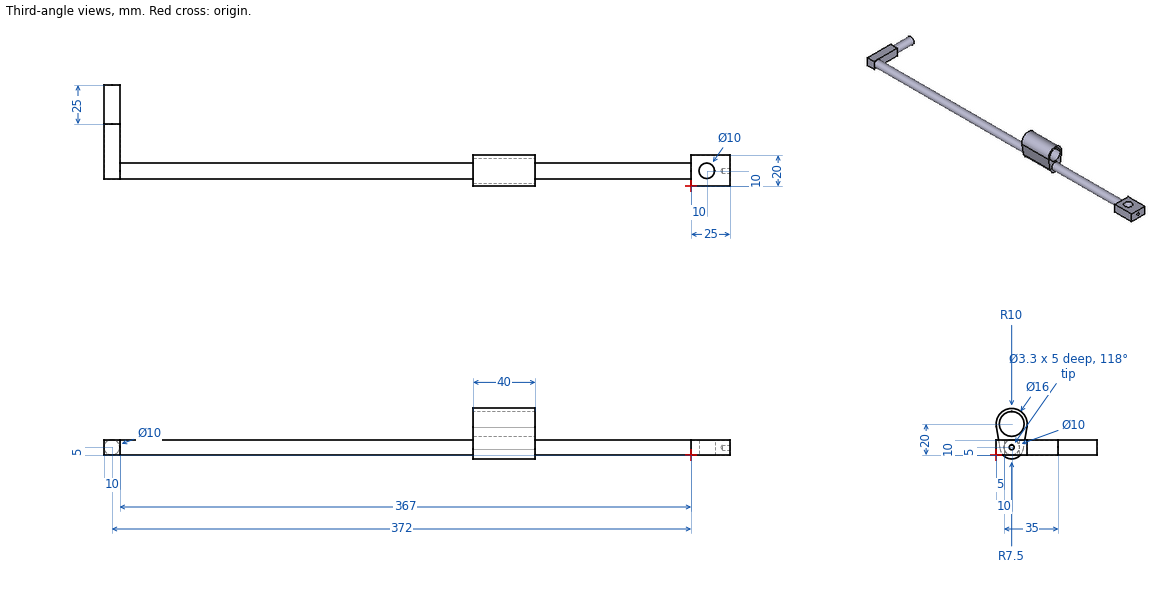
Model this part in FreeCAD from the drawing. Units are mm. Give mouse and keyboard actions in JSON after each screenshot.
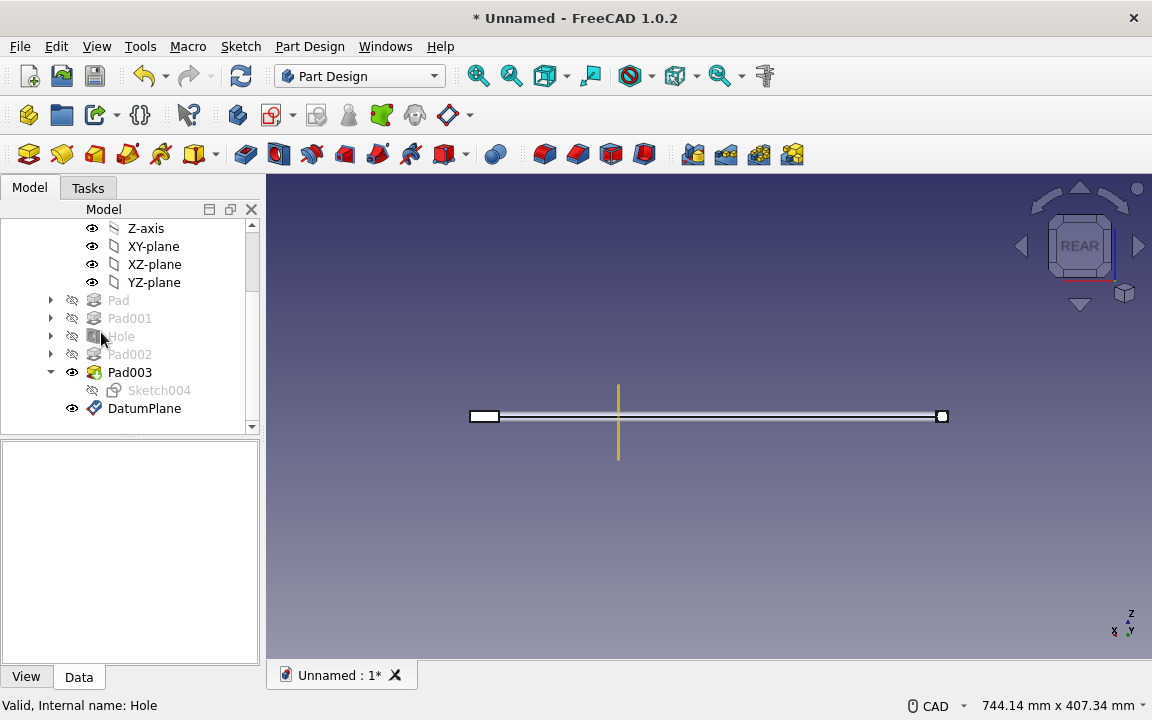
{"action": "left_click", "coordinate": [117, 408]}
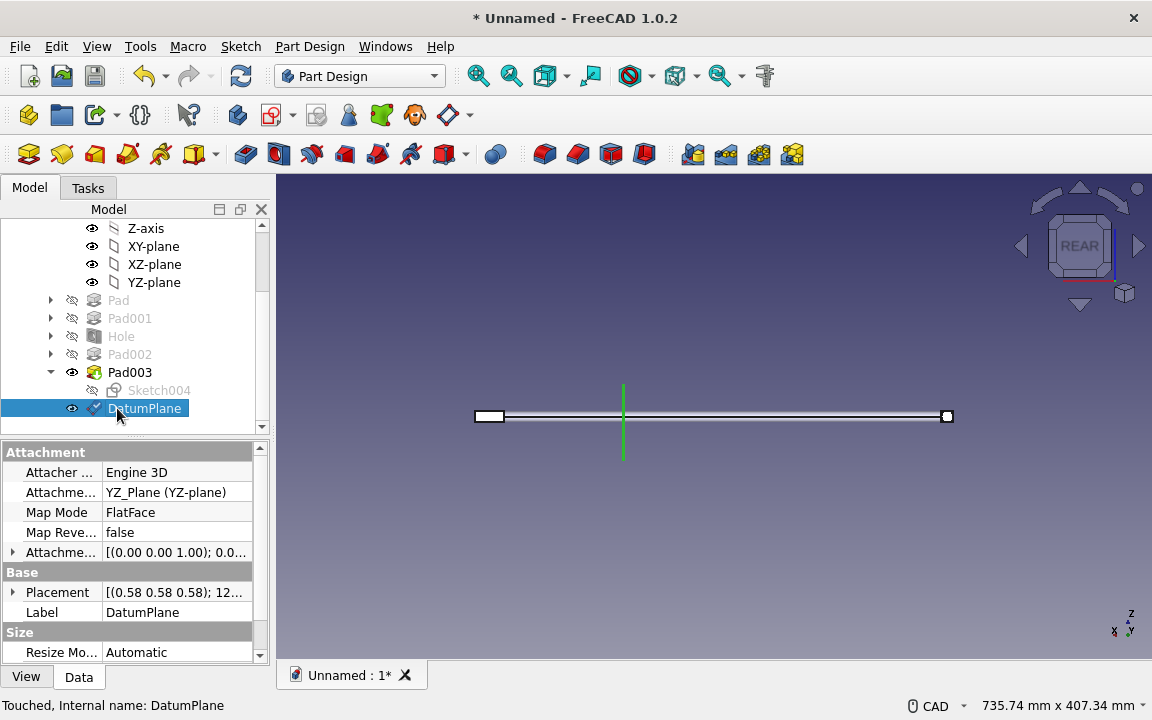
{"action": "left_click", "coordinate": [270, 116]}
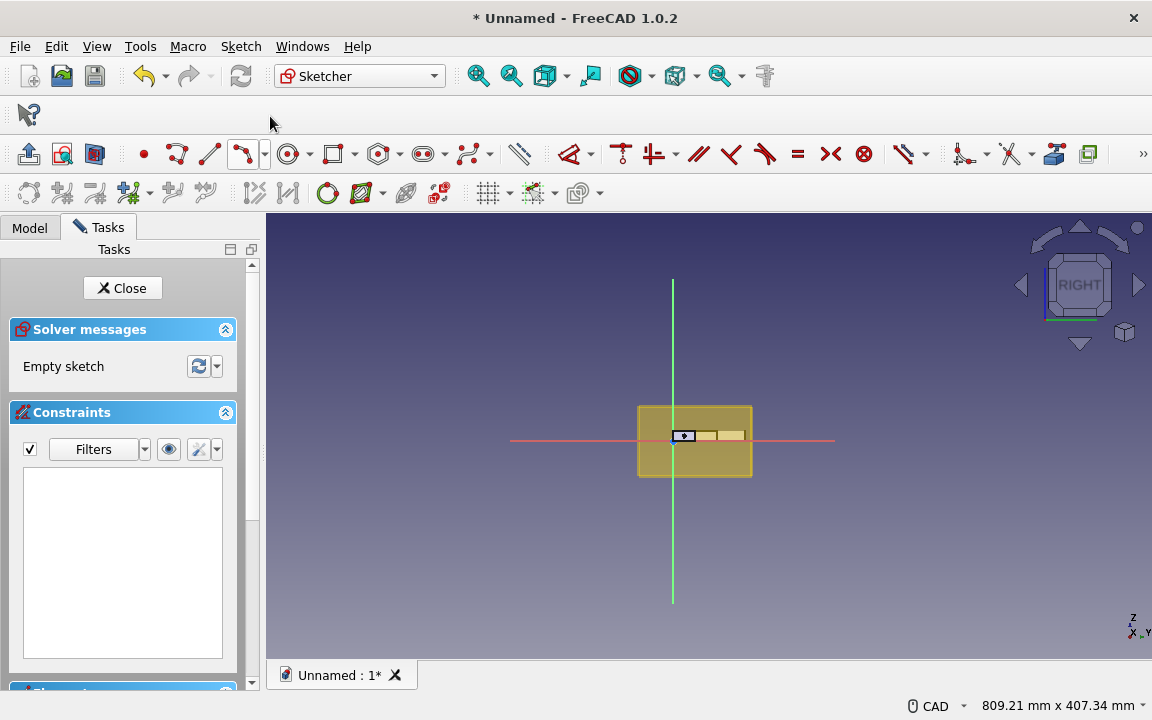
{"action": "key", "text": "q s"}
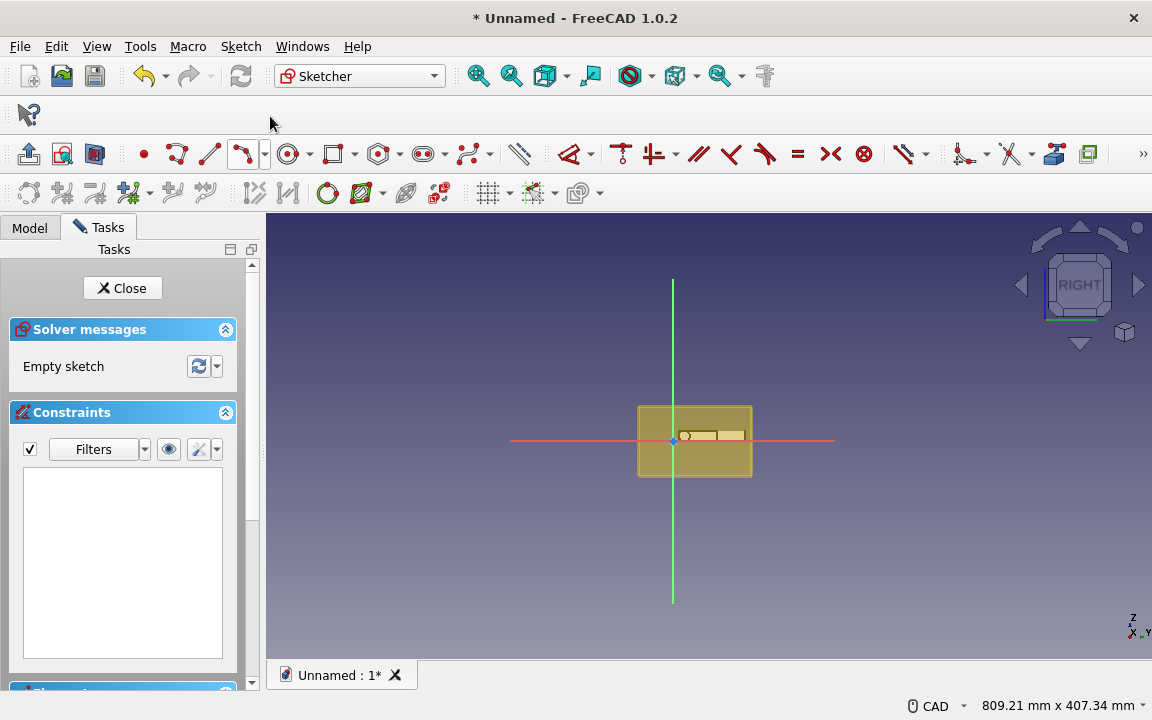
{"action": "scroll", "coordinate": [691, 425], "scroll_direction": "up", "scroll_amount": 10}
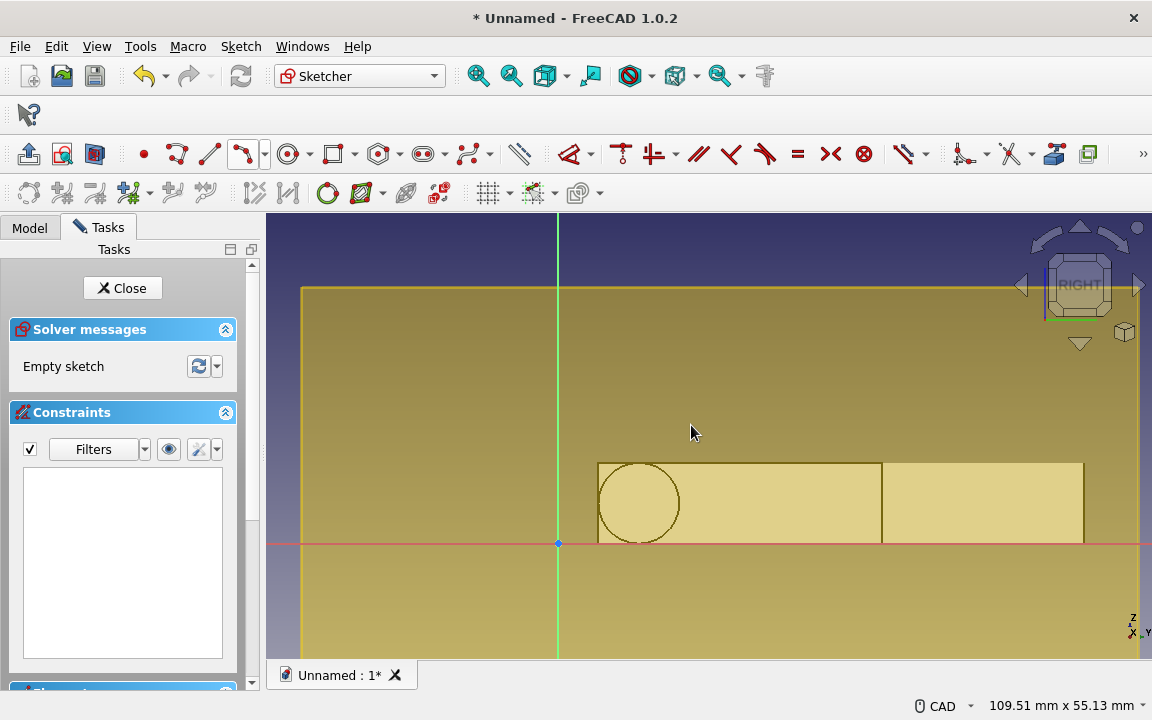
{"action": "left_click", "coordinate": [210, 154]}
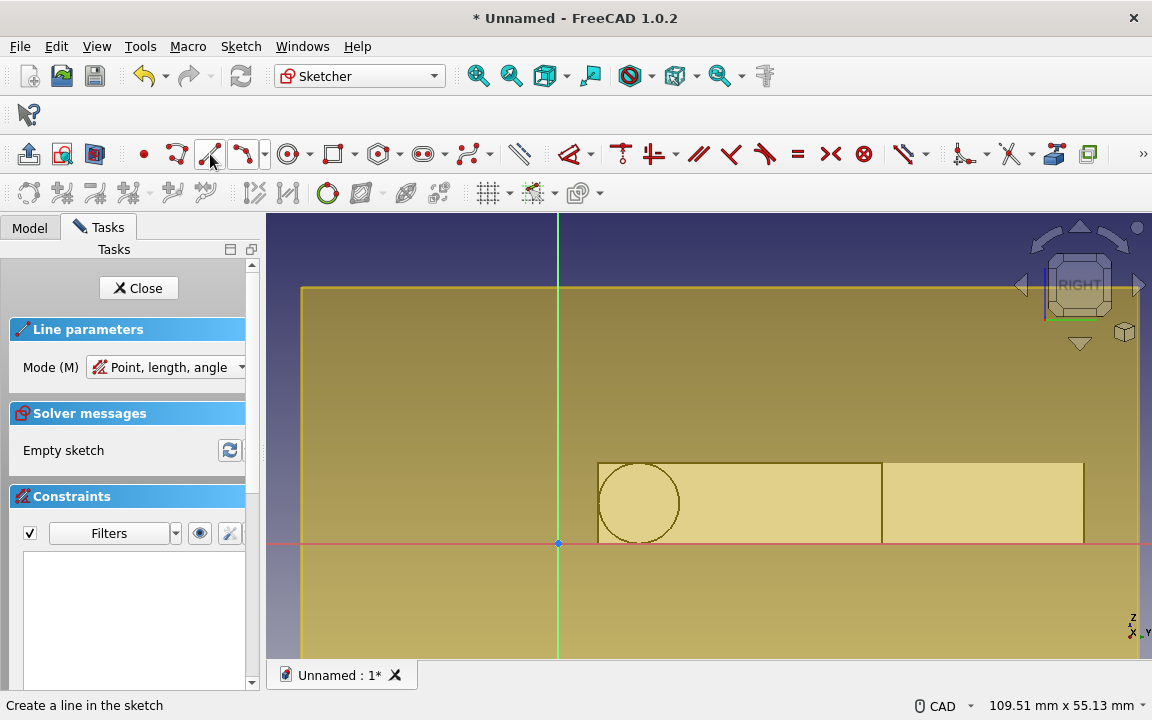
{"action": "left_click", "coordinate": [719, 395]}
{"action": "left_click", "coordinate": [699, 513]}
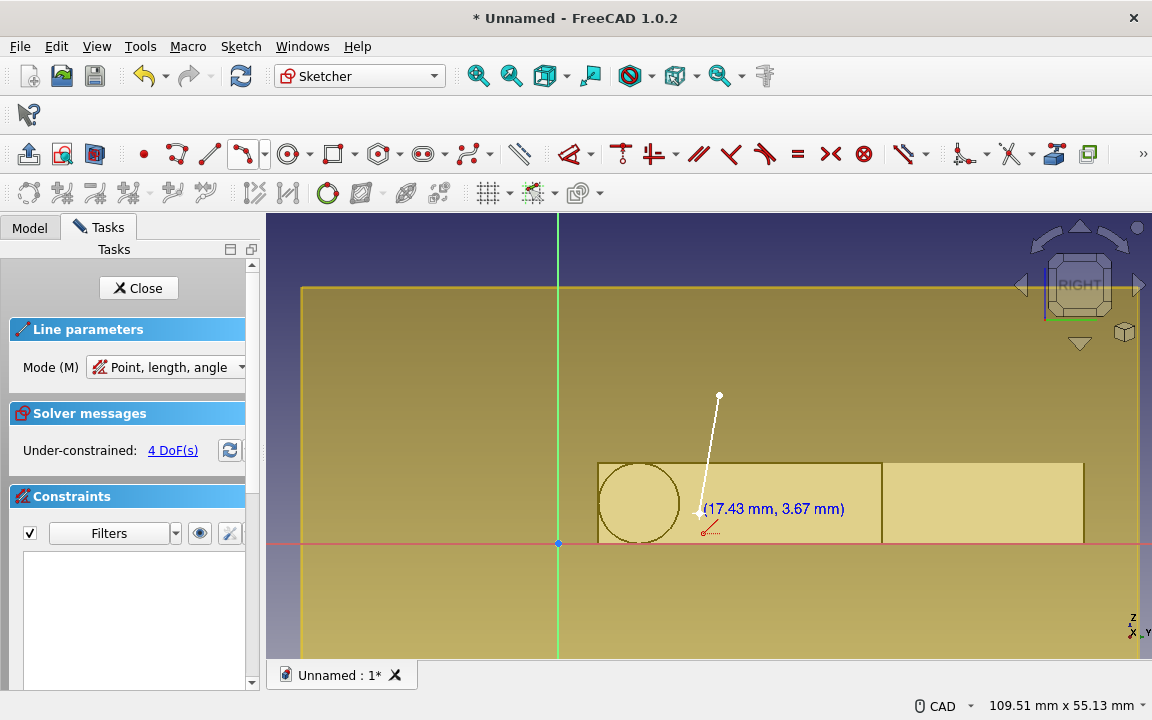
{"action": "left_click", "coordinate": [579, 513]}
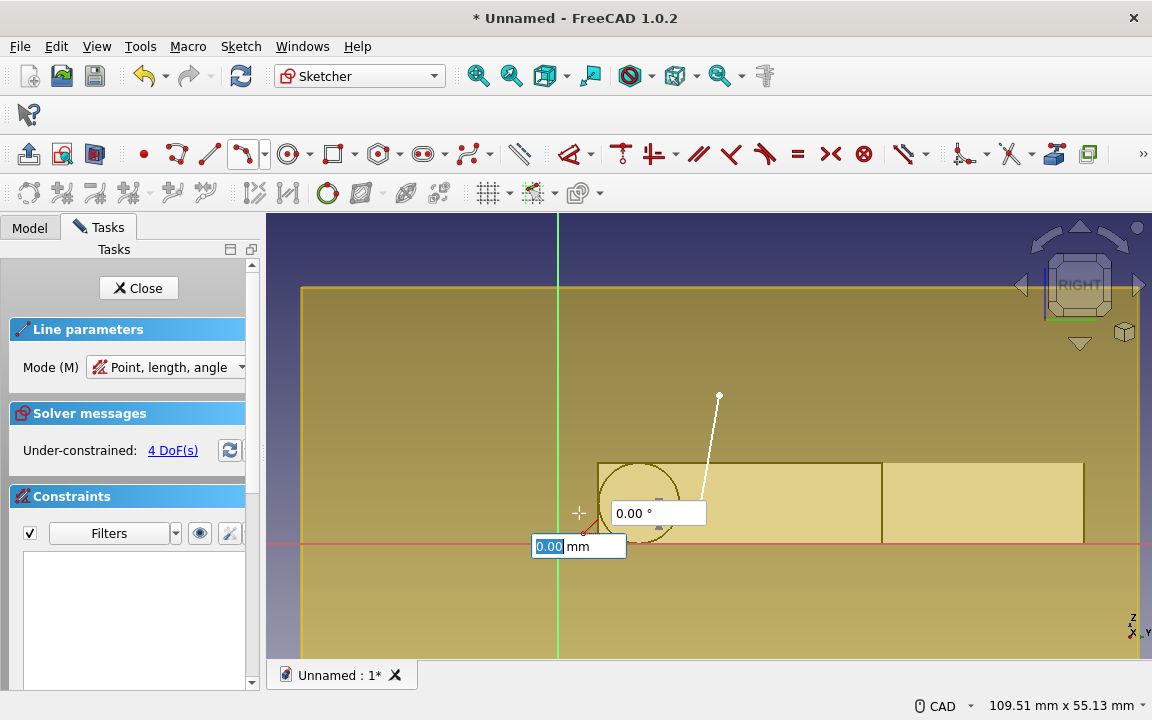
{"action": "scroll", "coordinate": [559, 395], "scroll_direction": "up", "scroll_amount": 14}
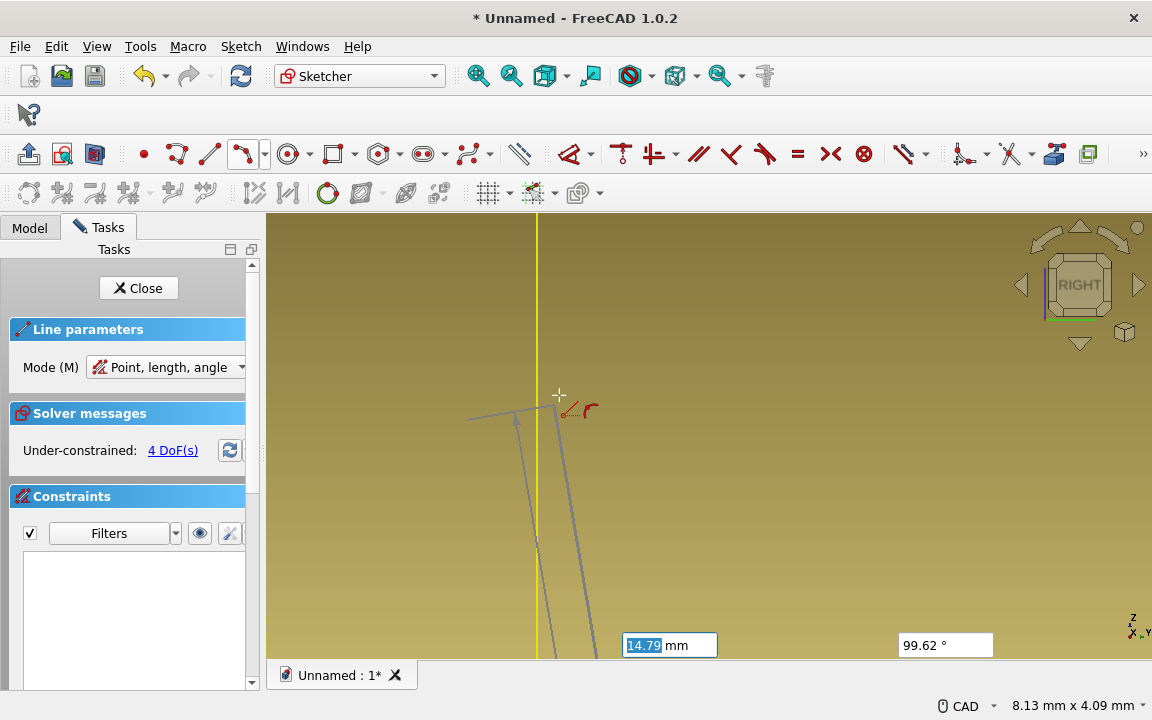
{"action": "left_click", "coordinate": [556, 395]}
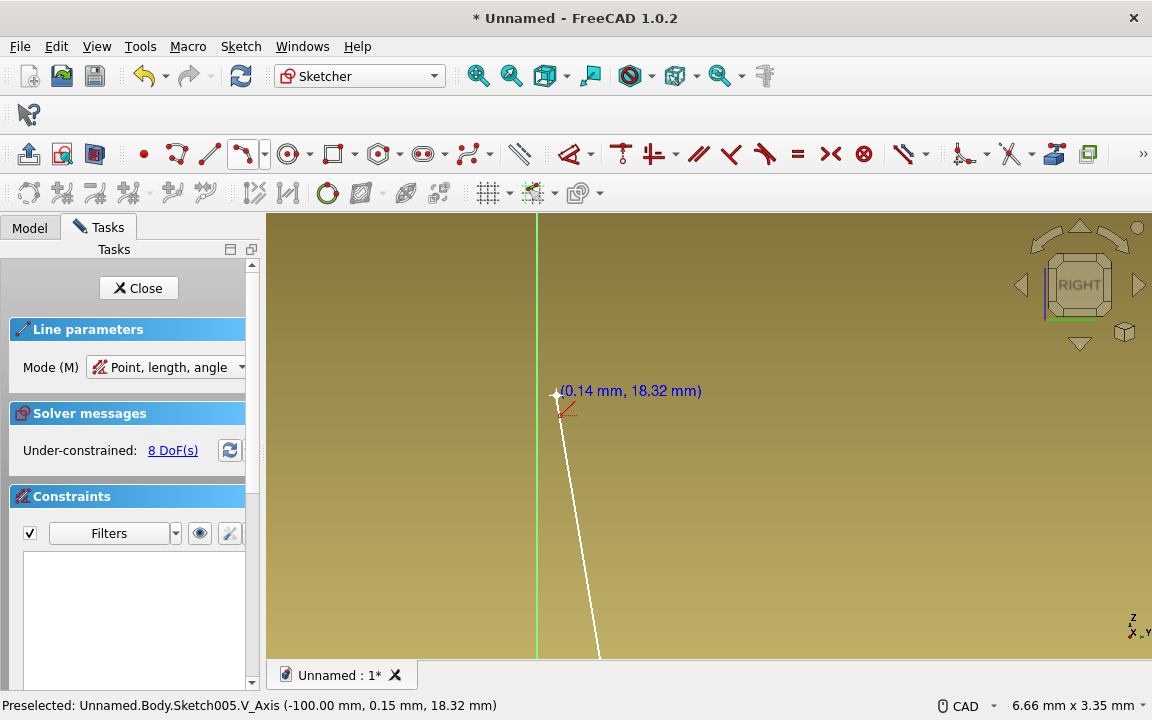
{"action": "left_click", "coordinate": [242, 154]}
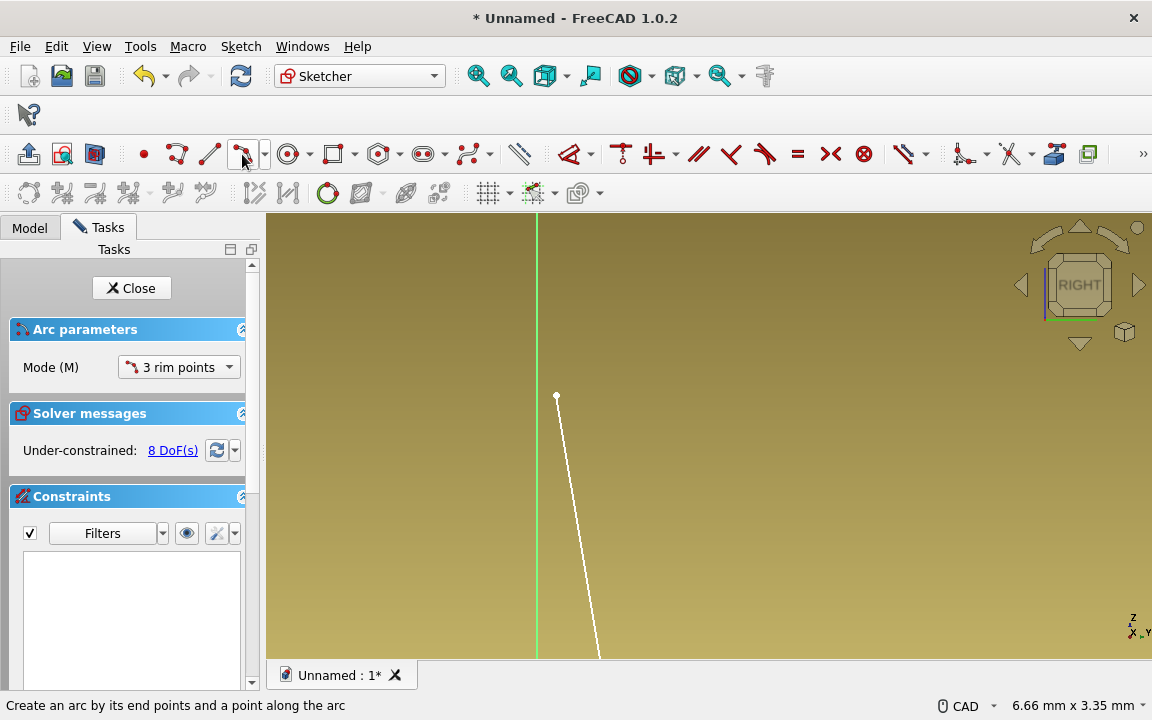
{"action": "scroll", "coordinate": [562, 399], "scroll_direction": "down", "scroll_amount": 14}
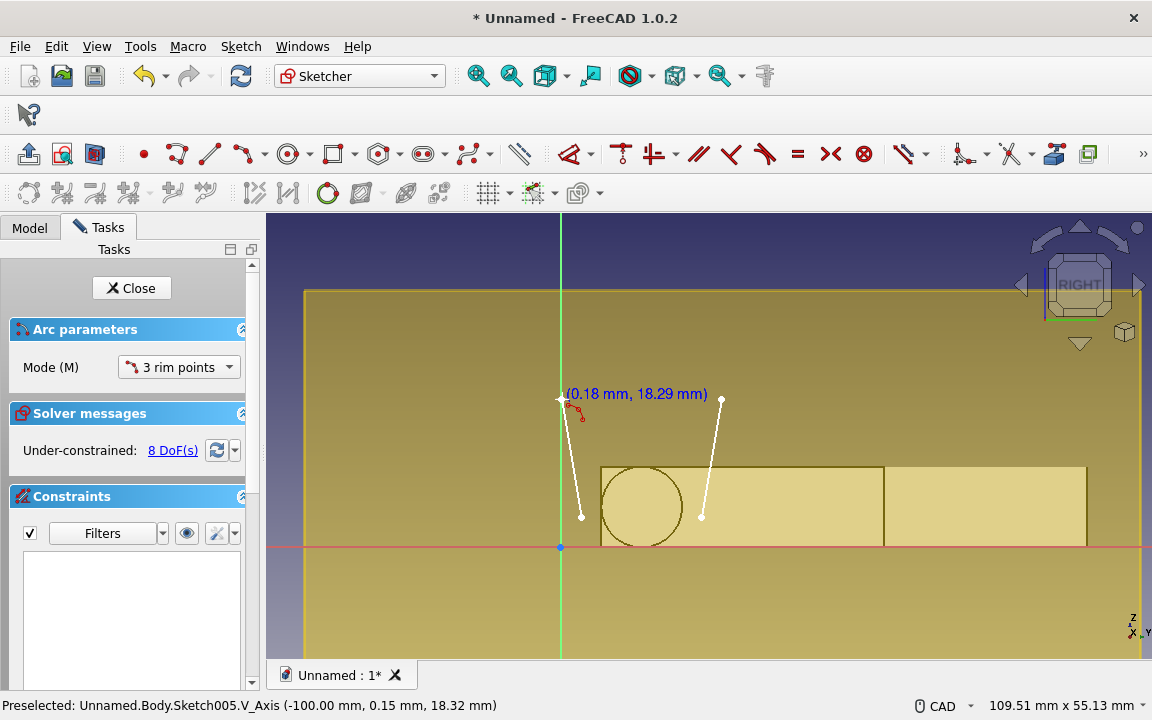
{"action": "left_click", "coordinate": [702, 518]}
{"action": "left_click", "coordinate": [582, 518]}
{"action": "left_click", "coordinate": [642, 568]}